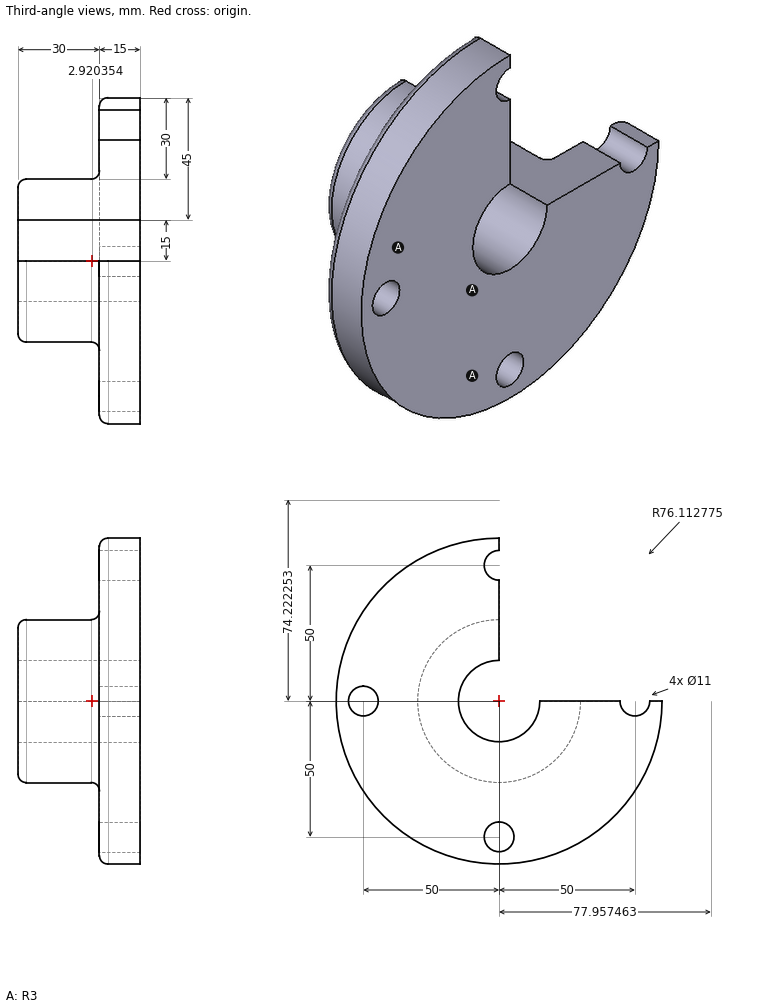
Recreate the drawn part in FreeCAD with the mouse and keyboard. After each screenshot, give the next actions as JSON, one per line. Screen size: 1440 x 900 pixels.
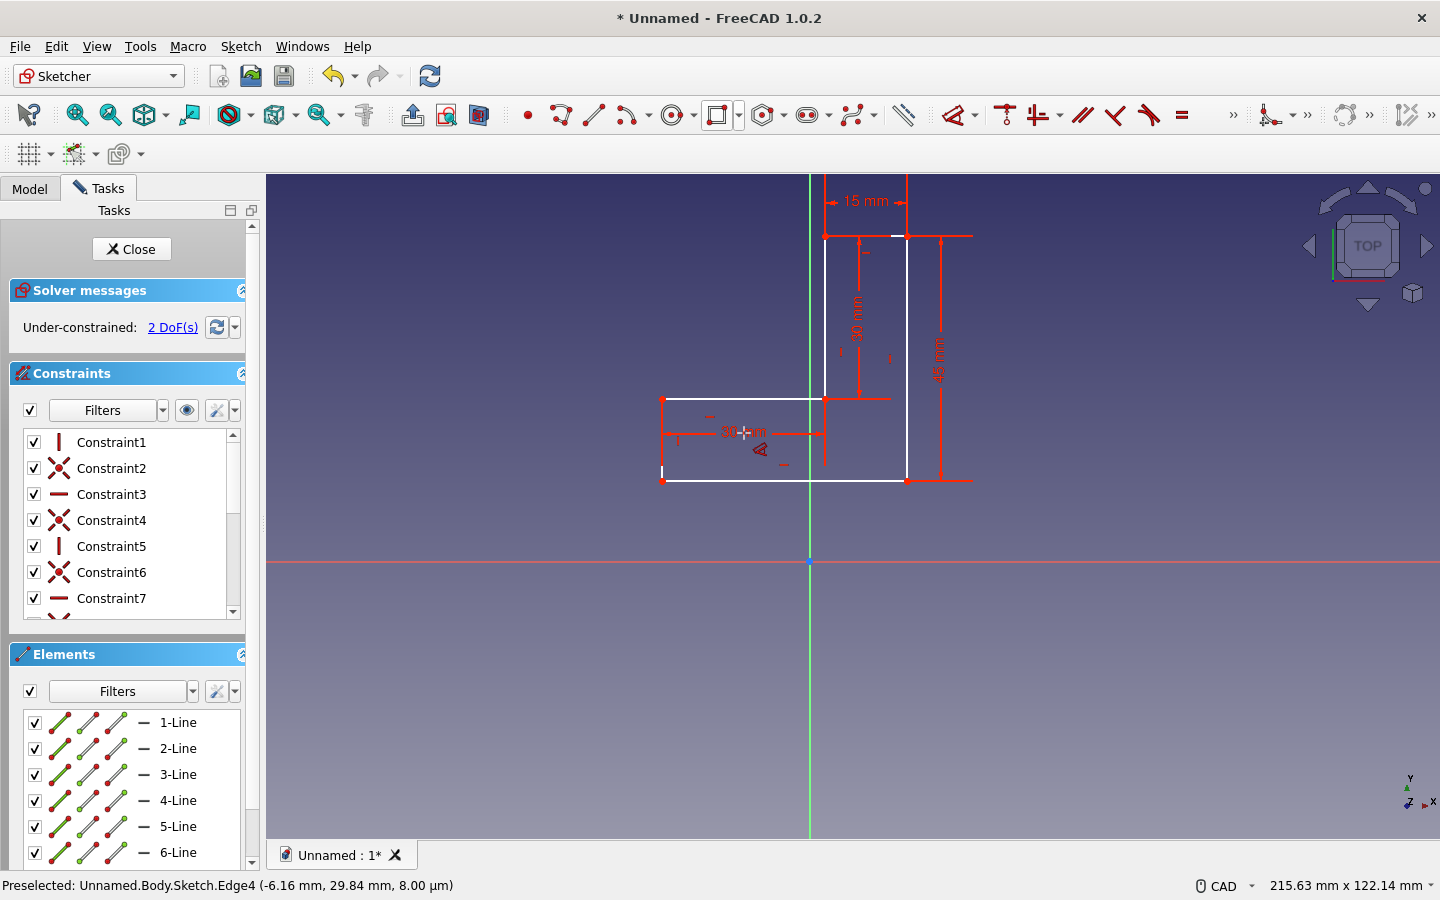
{"action": "left_click", "coordinate": [907, 481]}
{"action": "left_click", "coordinate": [941, 521]}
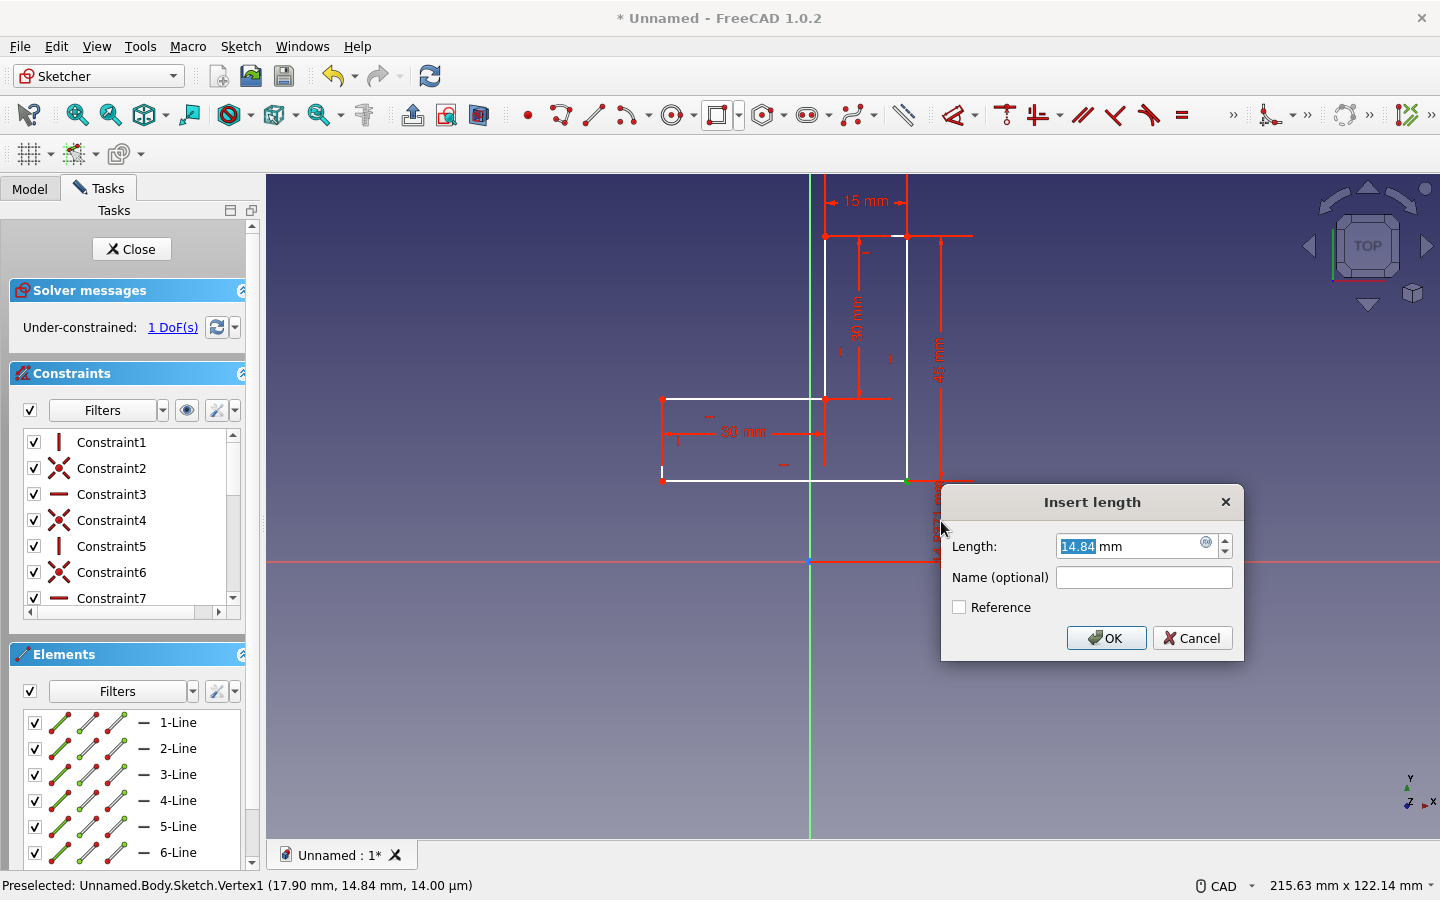
{"action": "type", "text": "15"}
{"action": "key", "text": "Return"}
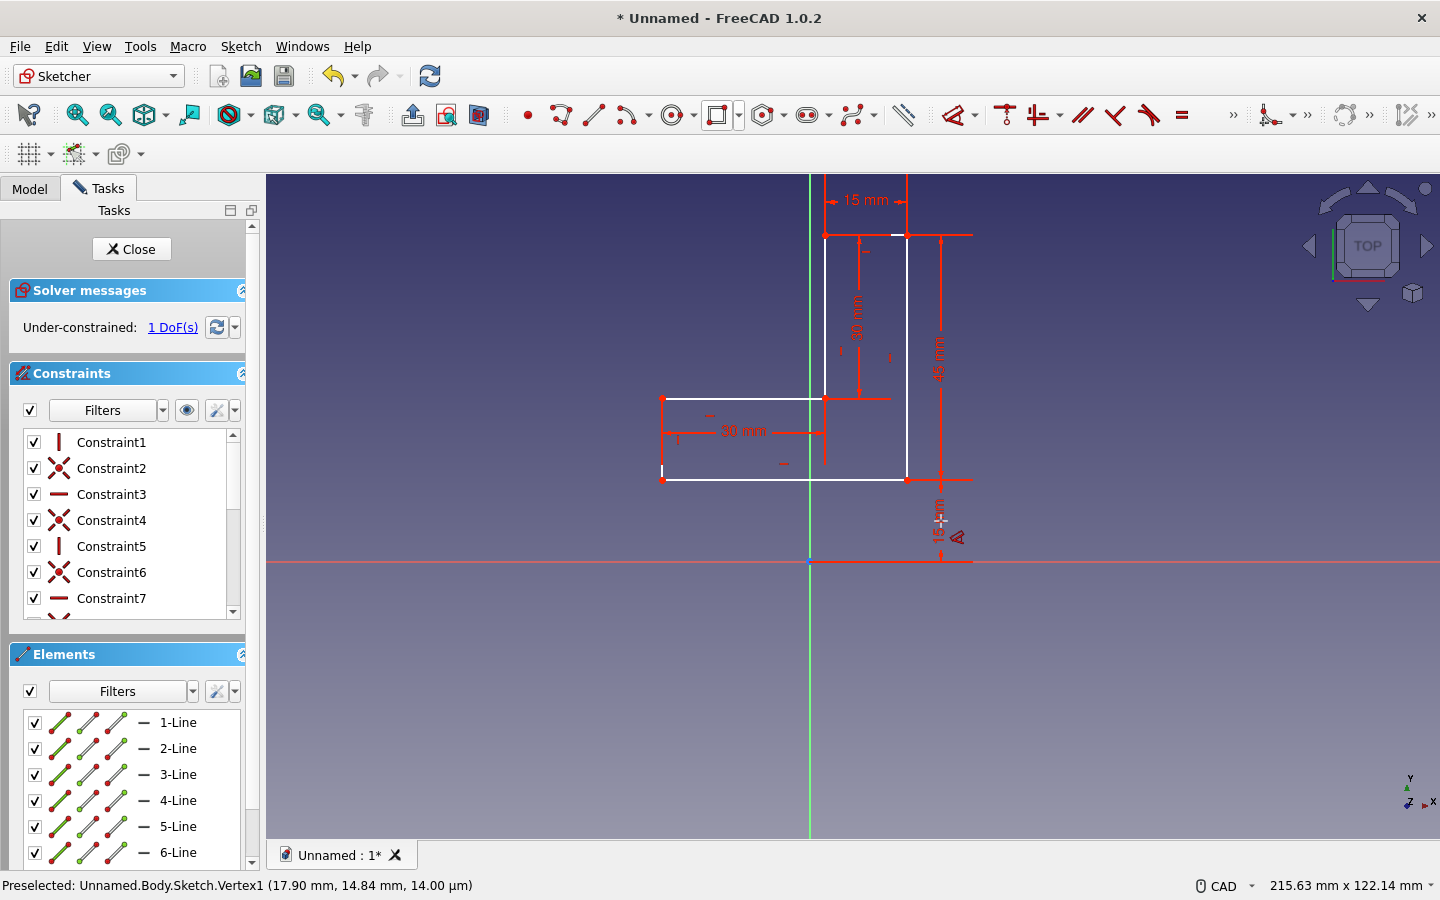
{"action": "scroll", "coordinate": [825, 235], "scroll_direction": "up", "scroll_amount": 5}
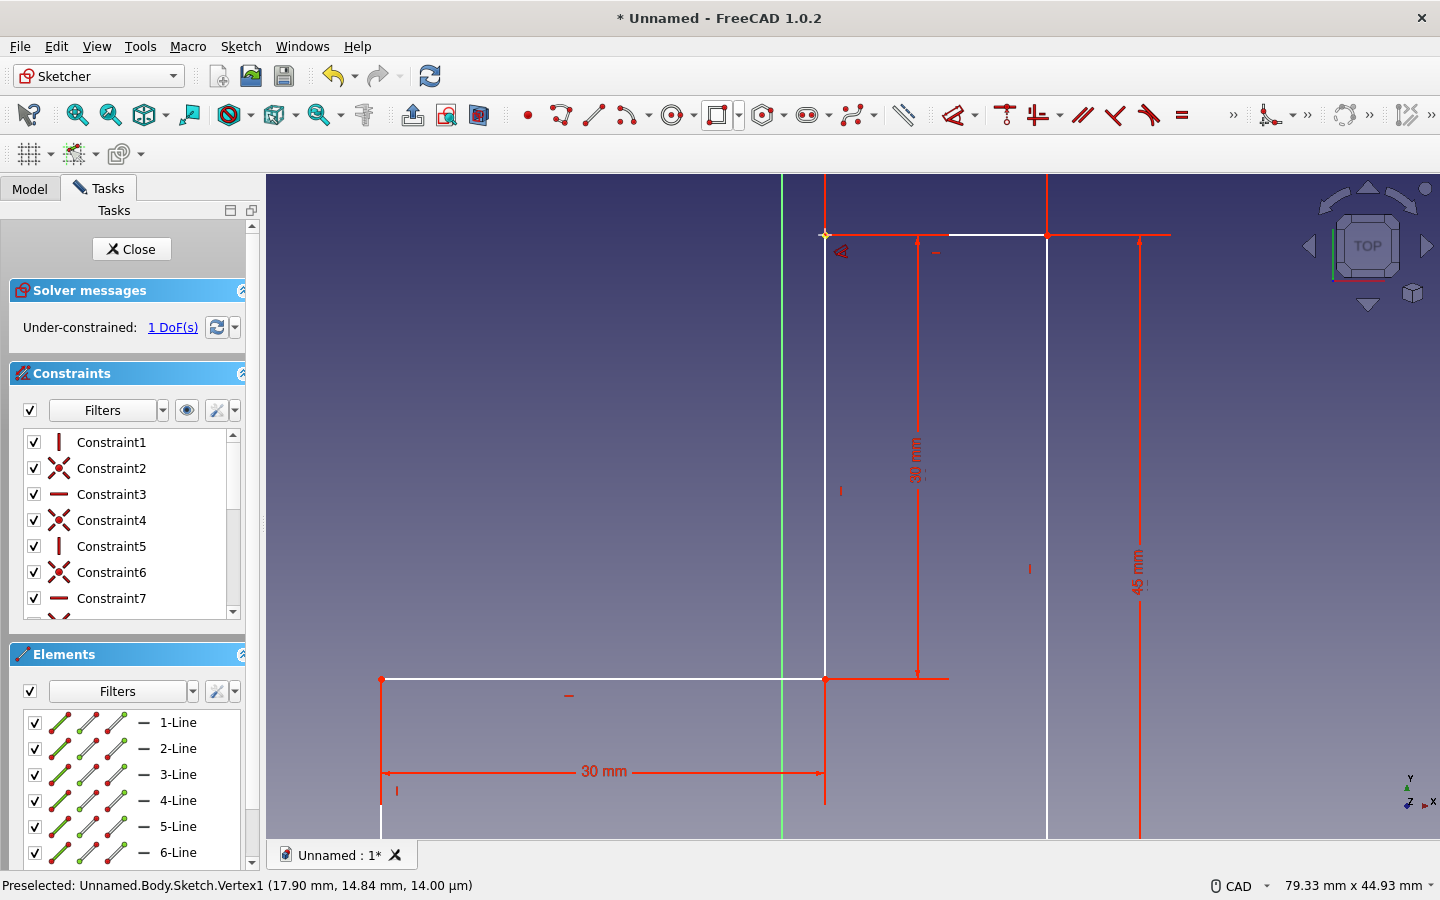
{"action": "left_click", "coordinate": [825, 235]}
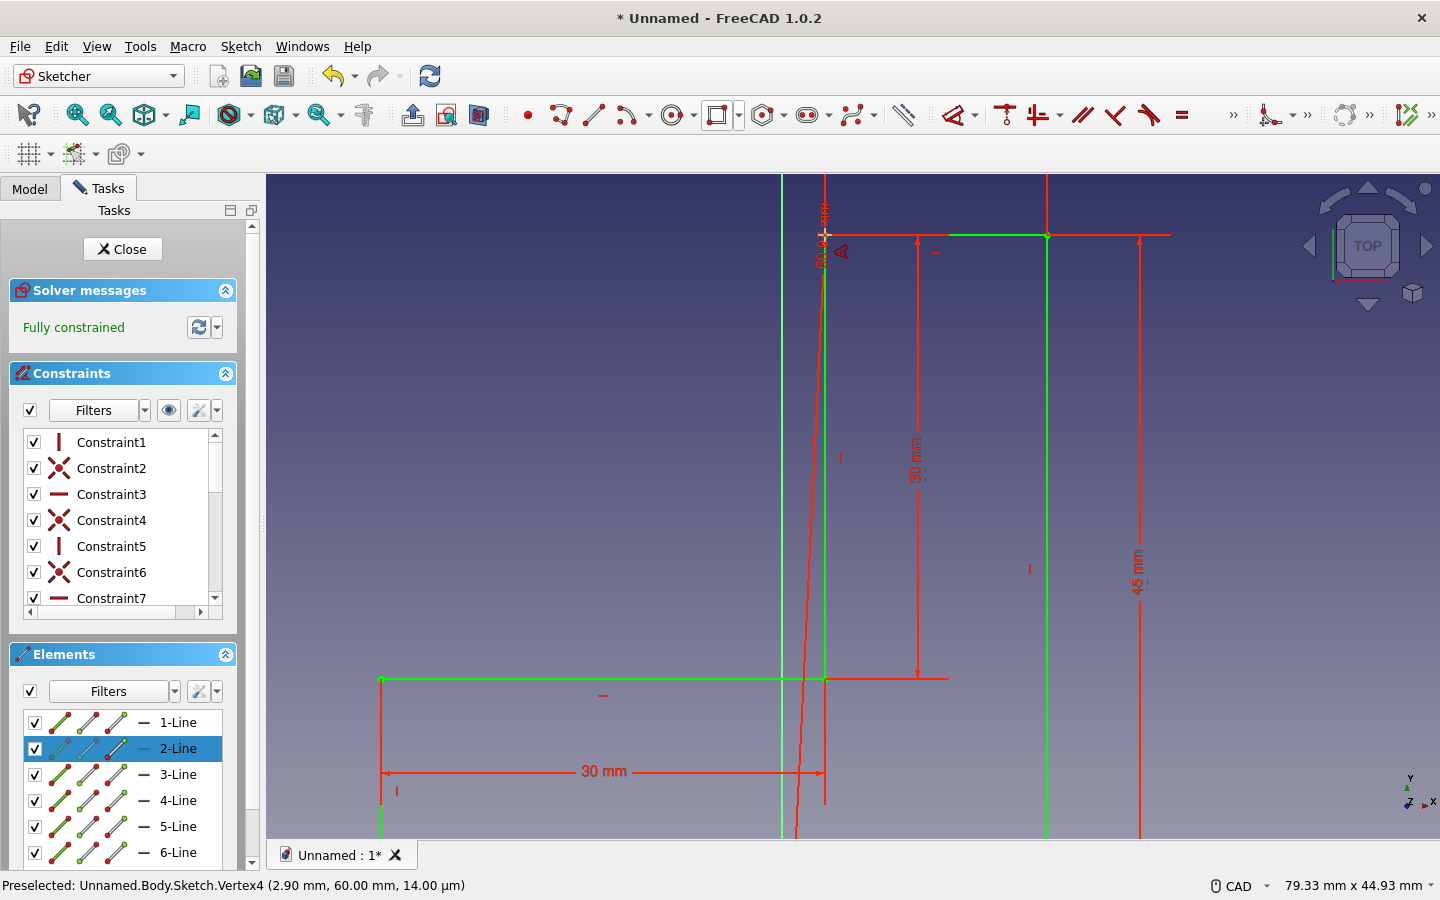
{"action": "key", "text": "Escape"}
{"action": "key", "text": "Escape"}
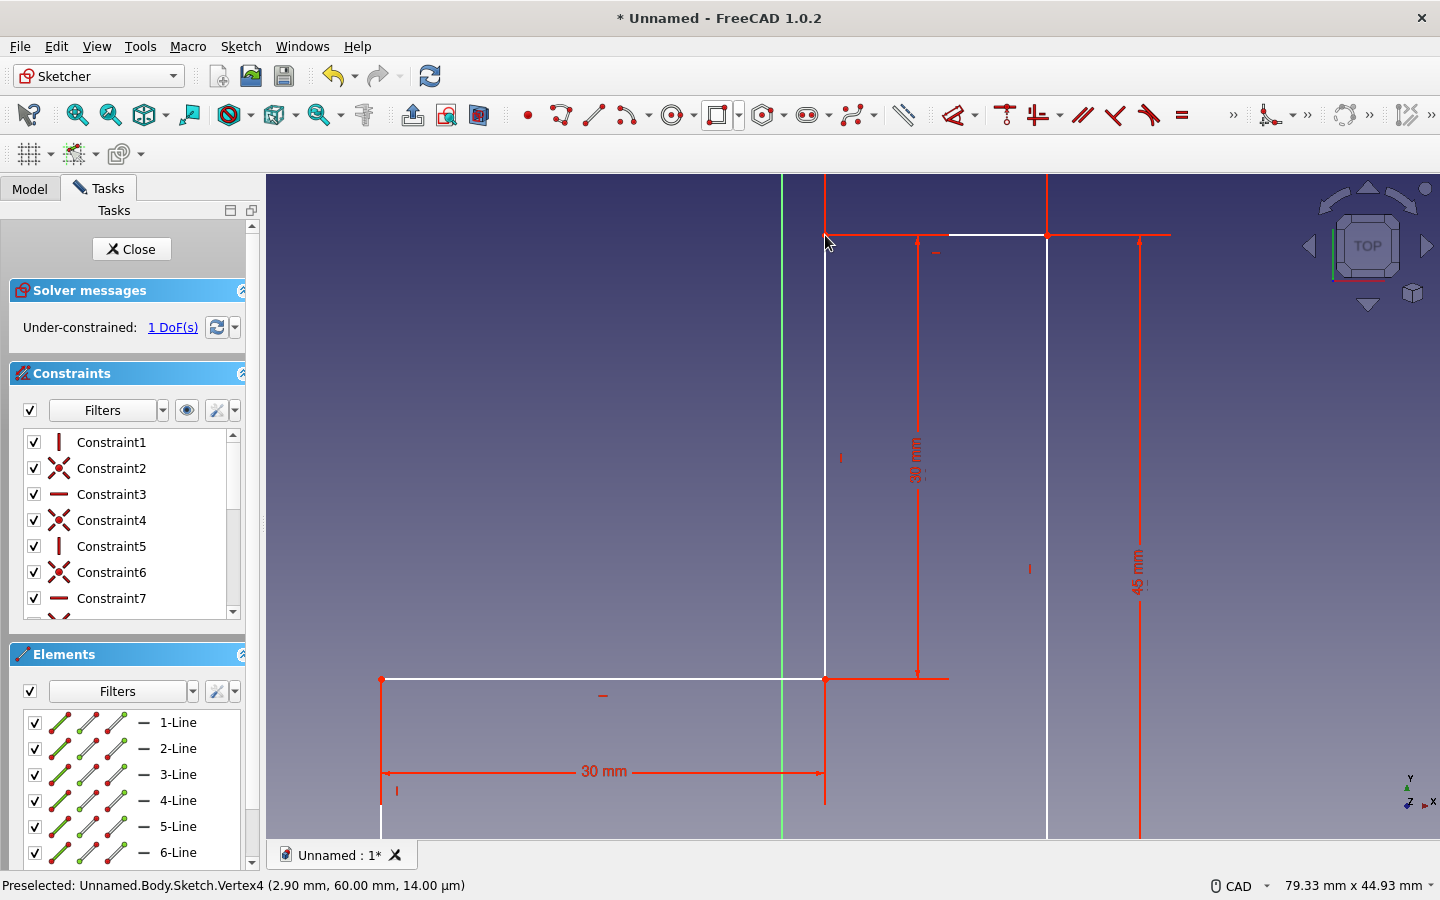
{"action": "left_click", "coordinate": [825, 235]}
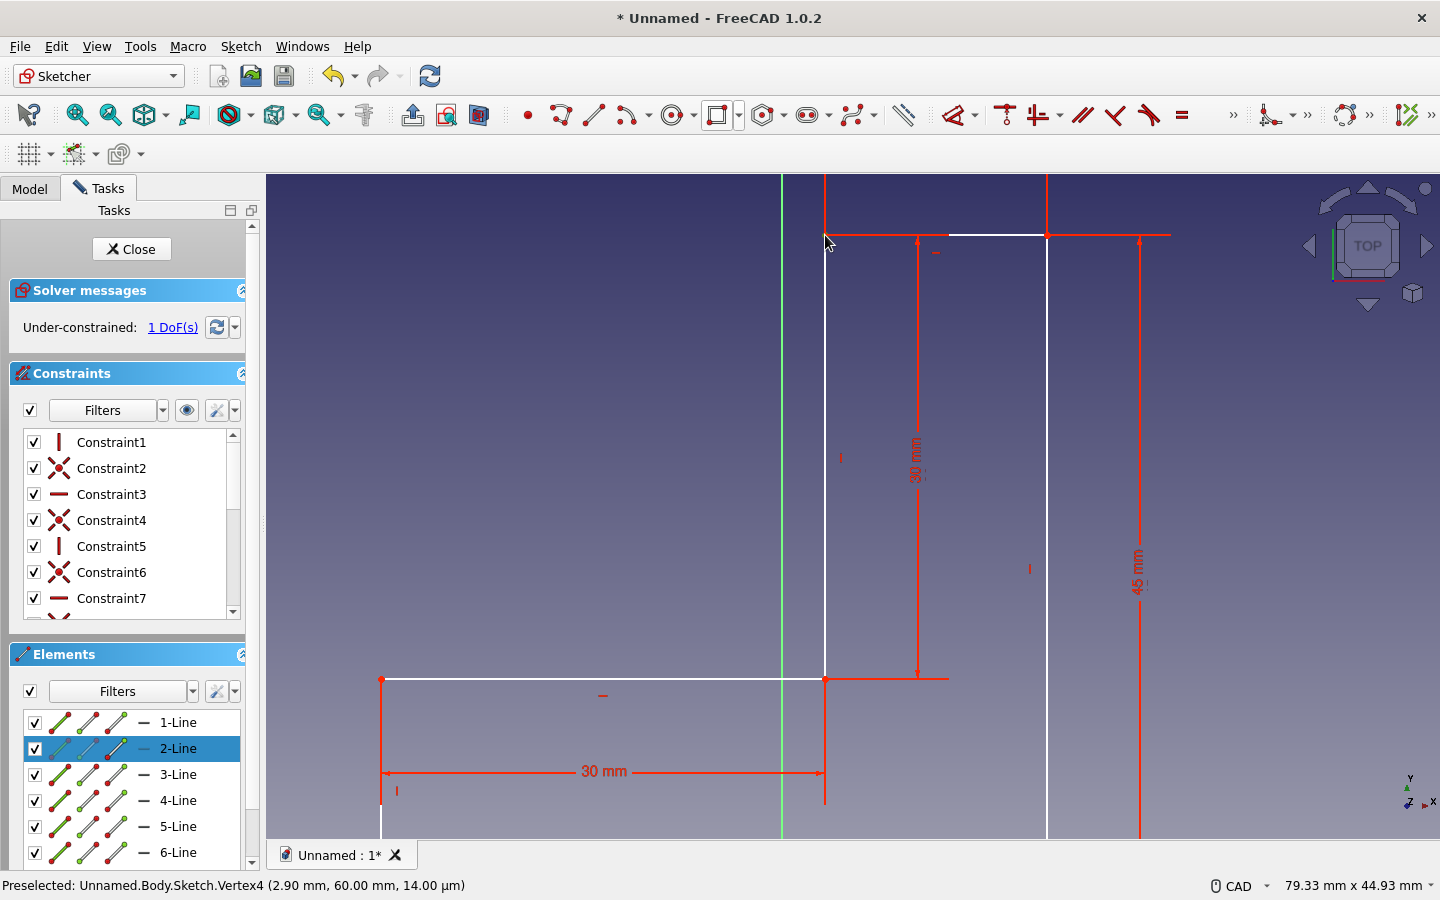
{"action": "left_click", "coordinate": [974, 116]}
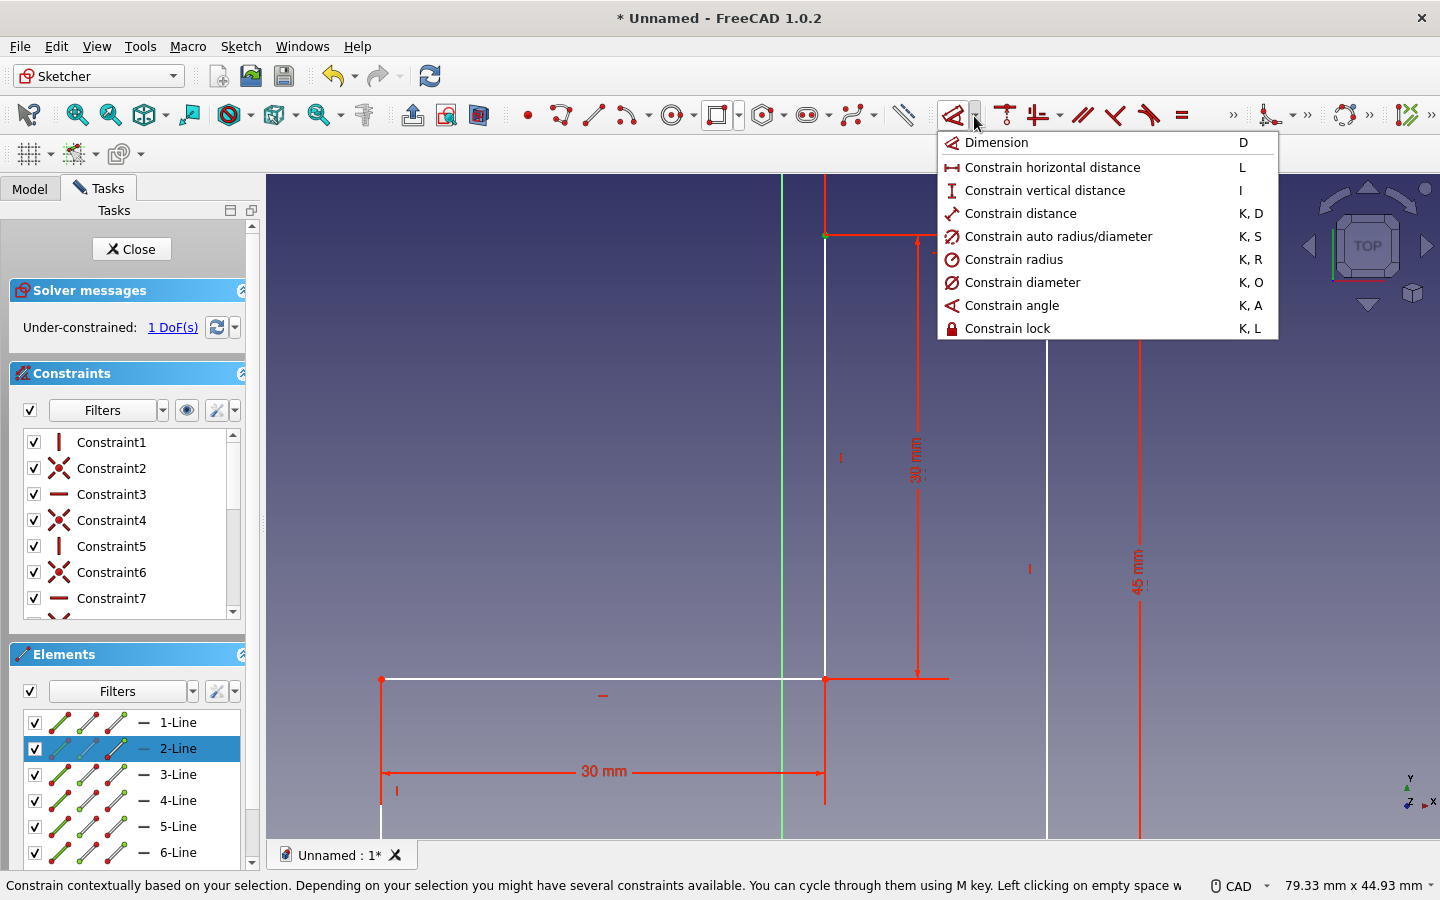
{"action": "left_click", "coordinate": [1108, 168]}